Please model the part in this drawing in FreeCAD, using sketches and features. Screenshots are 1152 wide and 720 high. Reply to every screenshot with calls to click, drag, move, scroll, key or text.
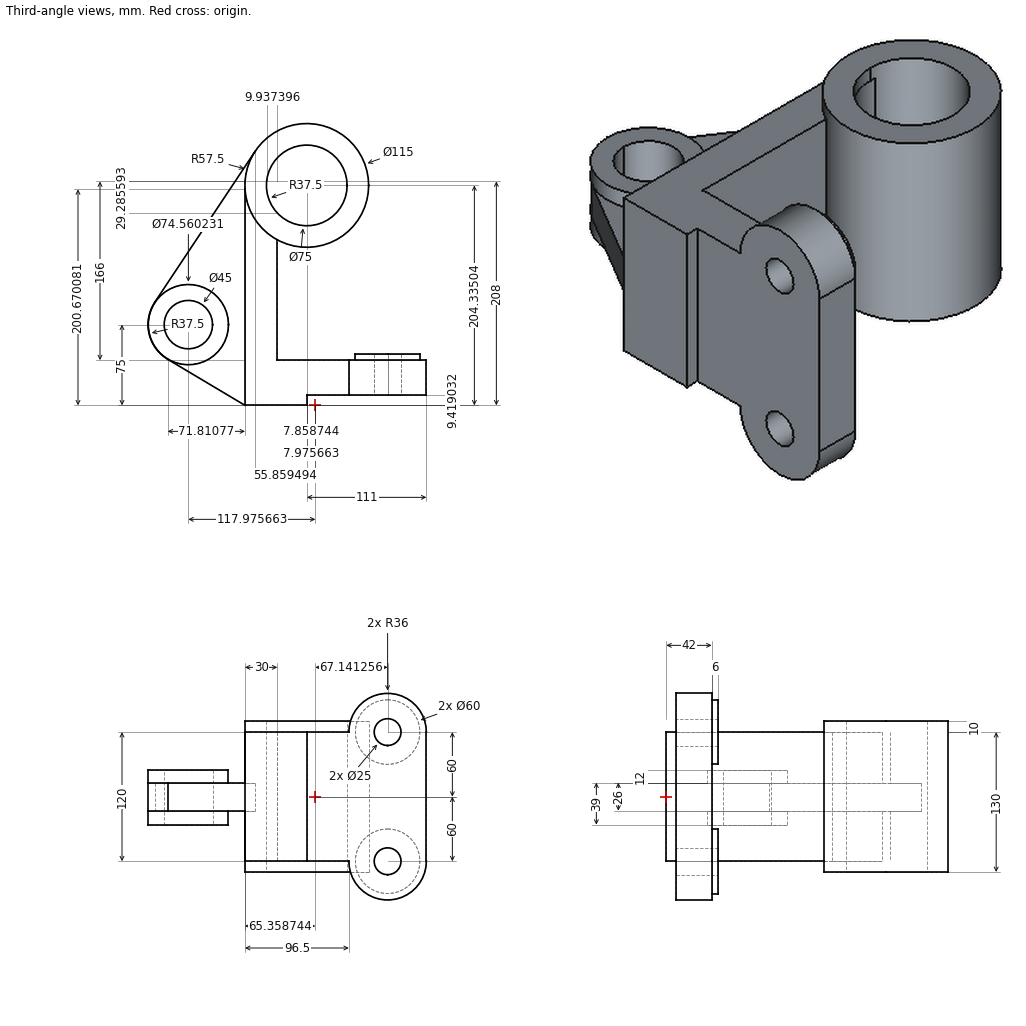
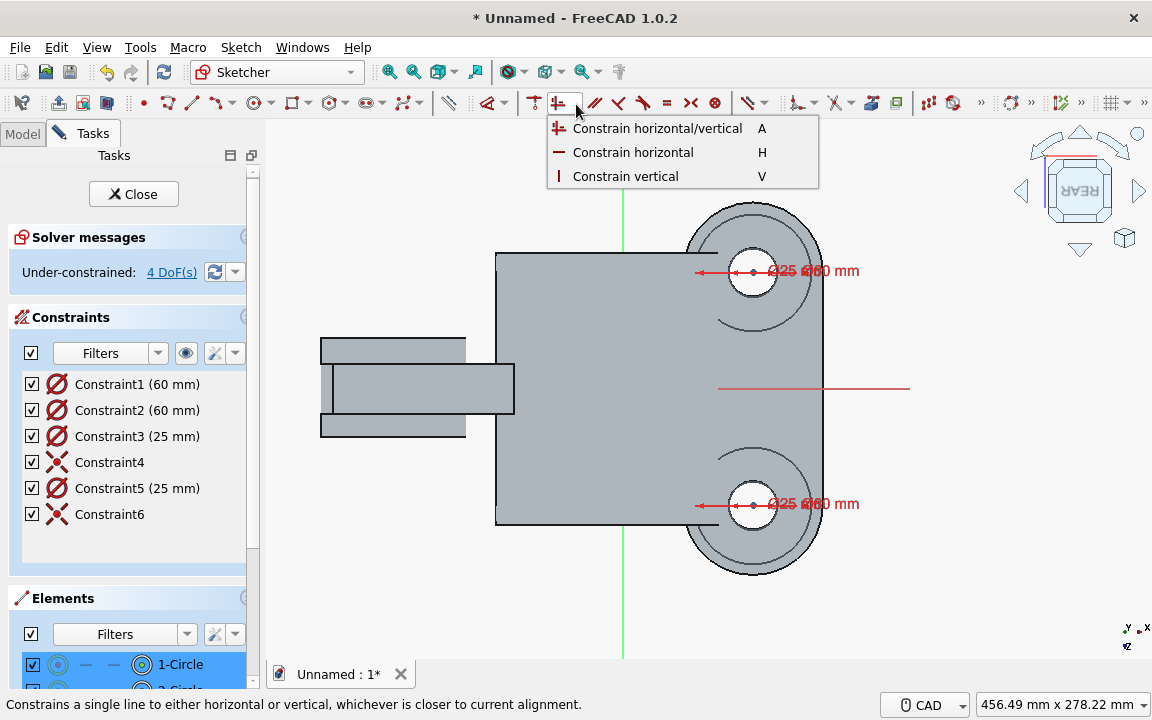
click(683, 176)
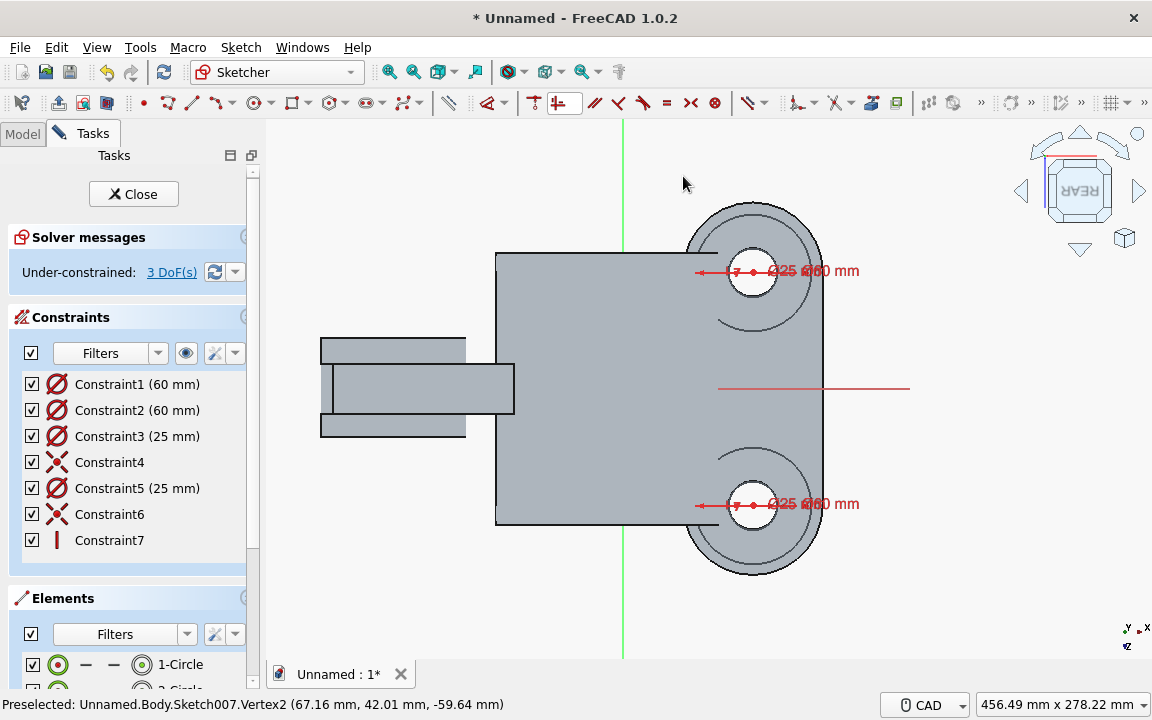
click(488, 104)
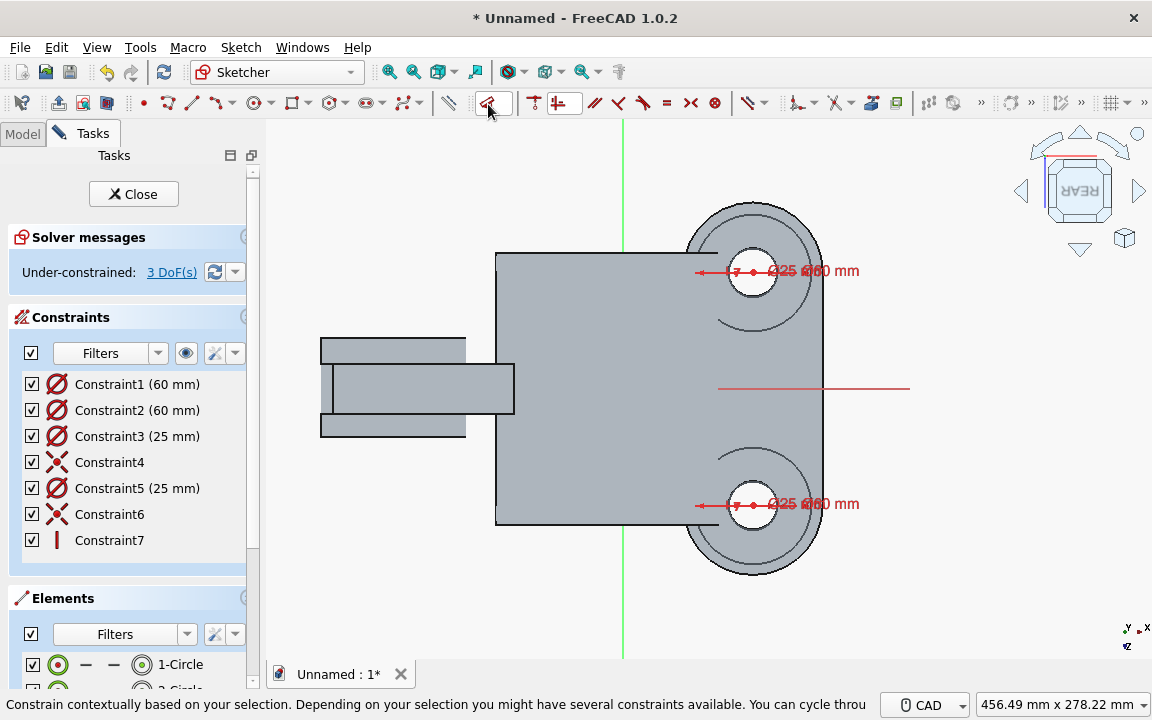
click(753, 506)
click(589, 447)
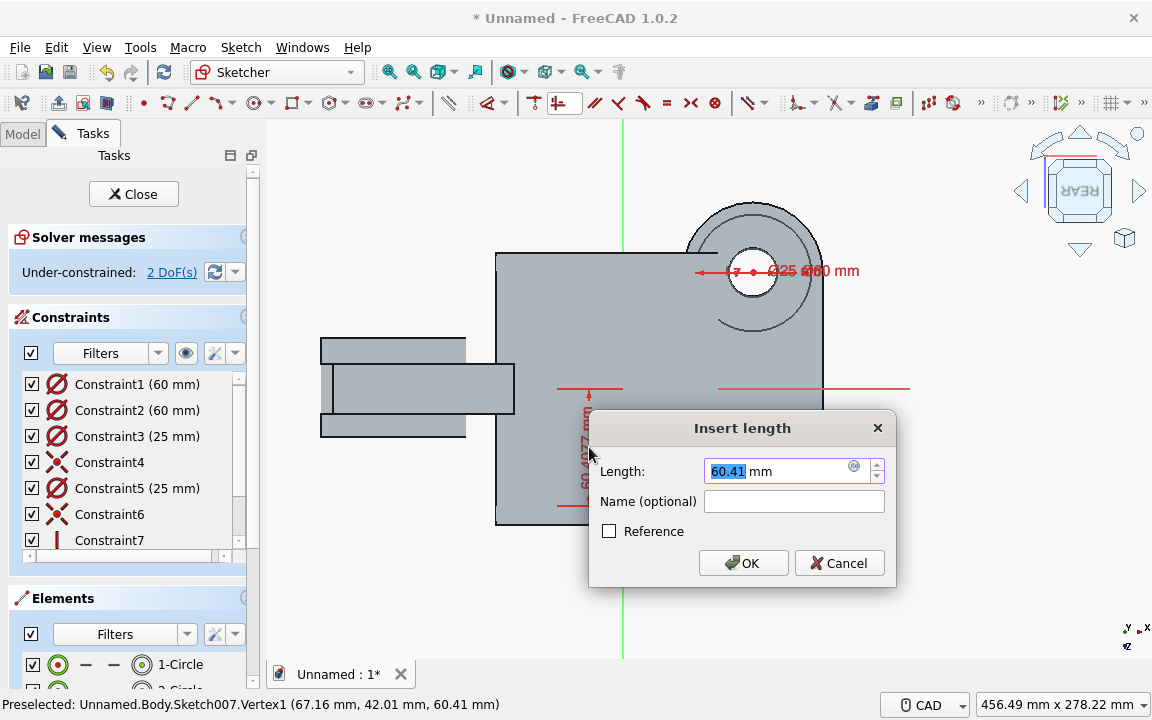
text(60)
key(Return)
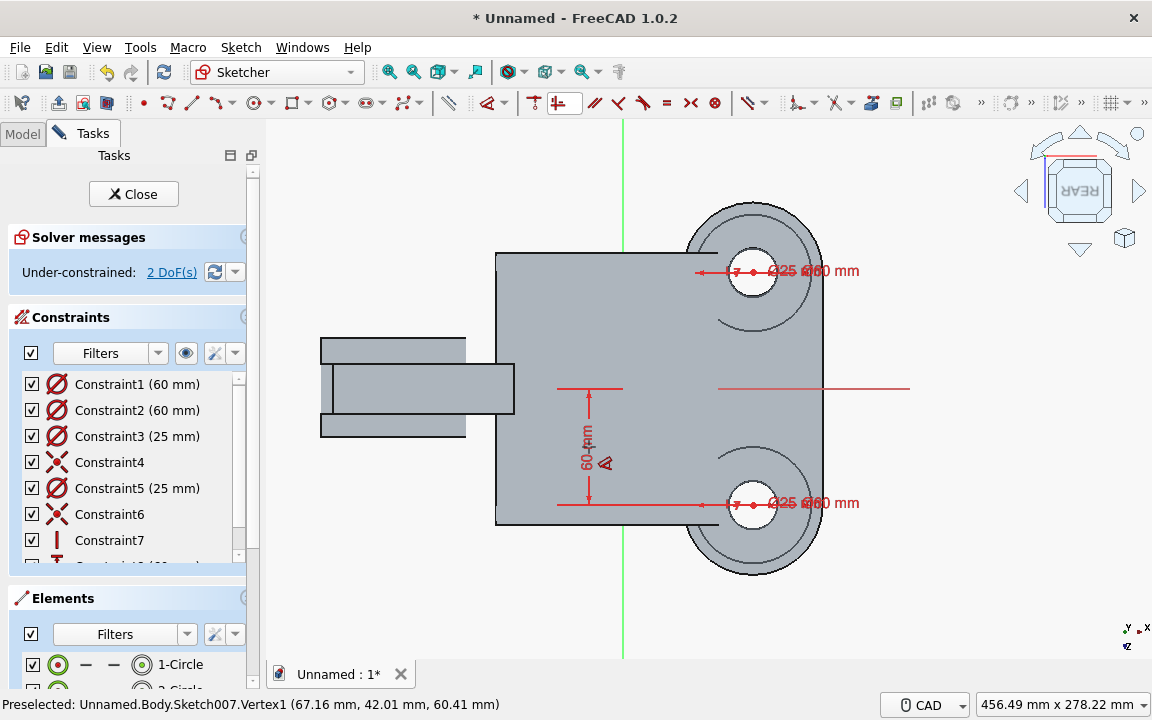
click(753, 273)
click(589, 331)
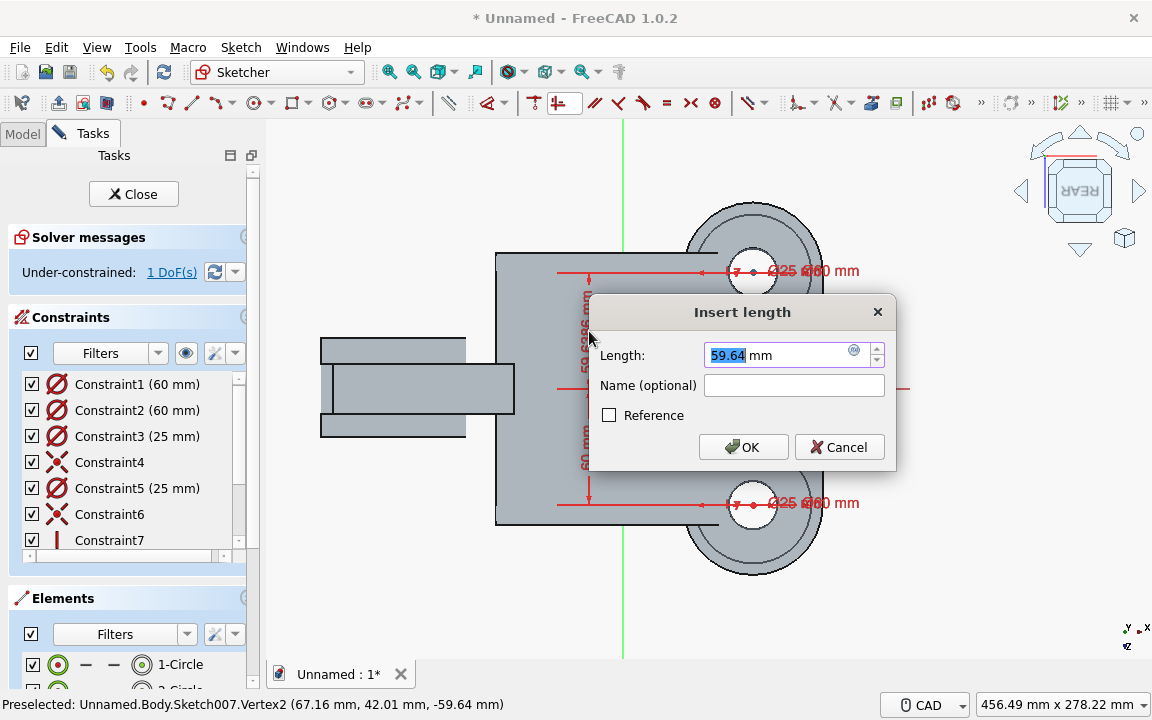
text(60)
key(Return)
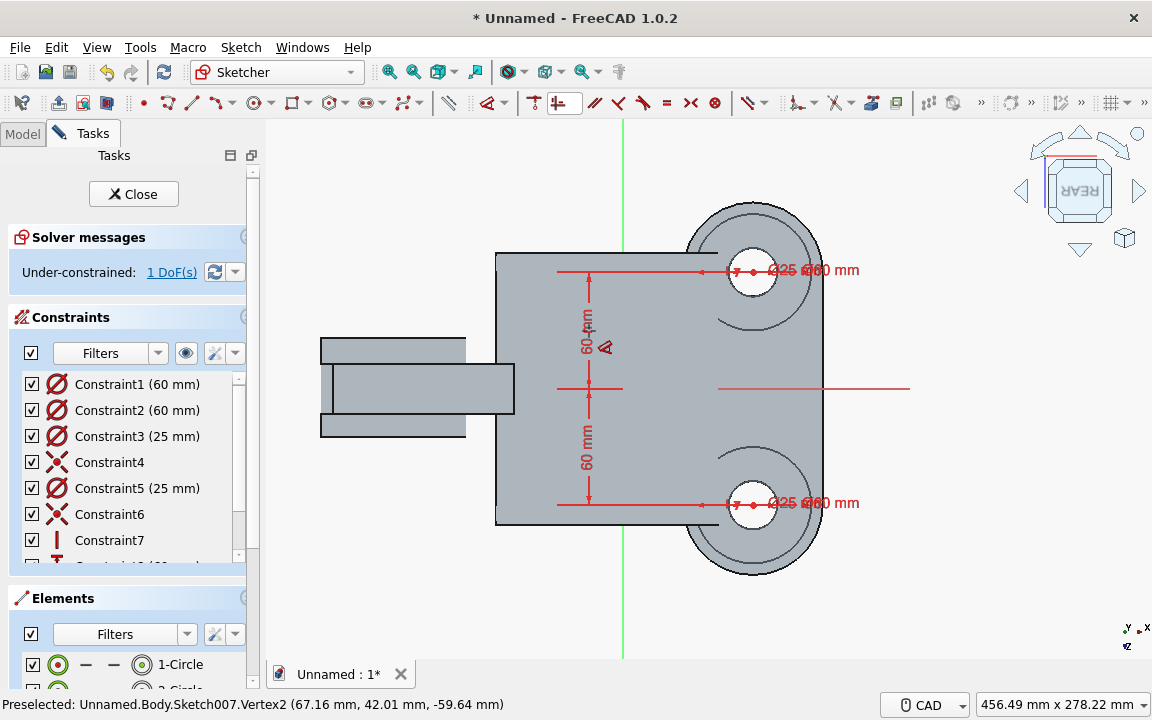
click(753, 505)
click(688, 539)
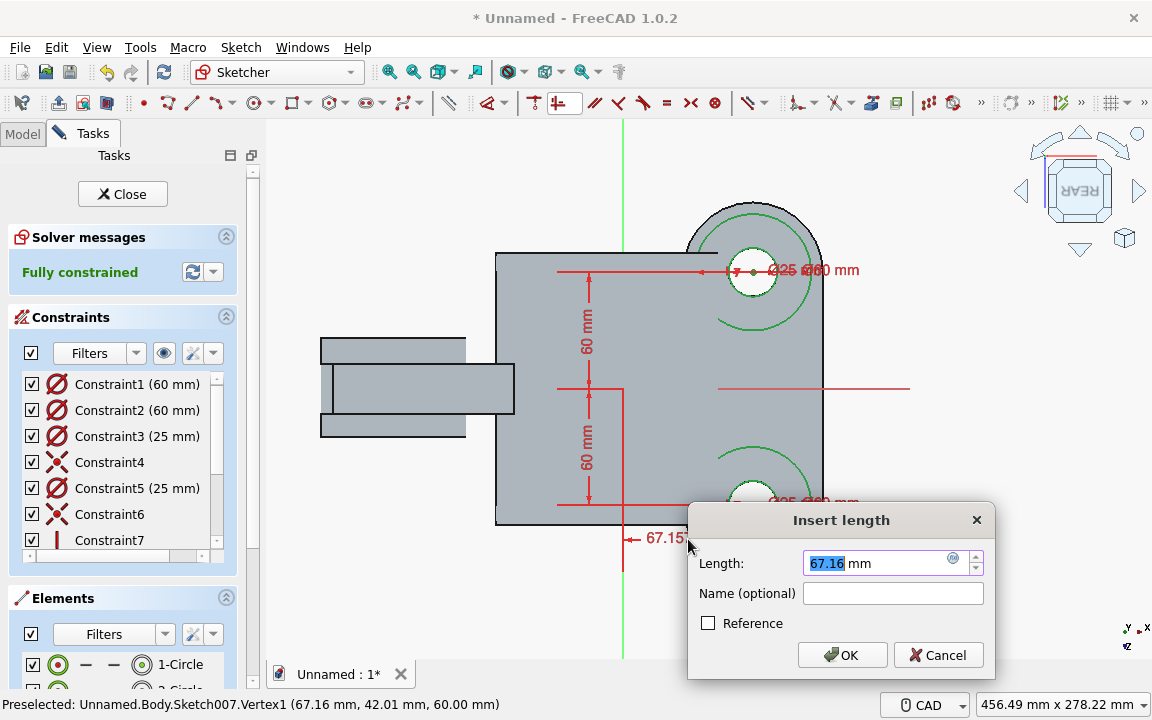
text(67.141256)
key(Return)
key(Escape)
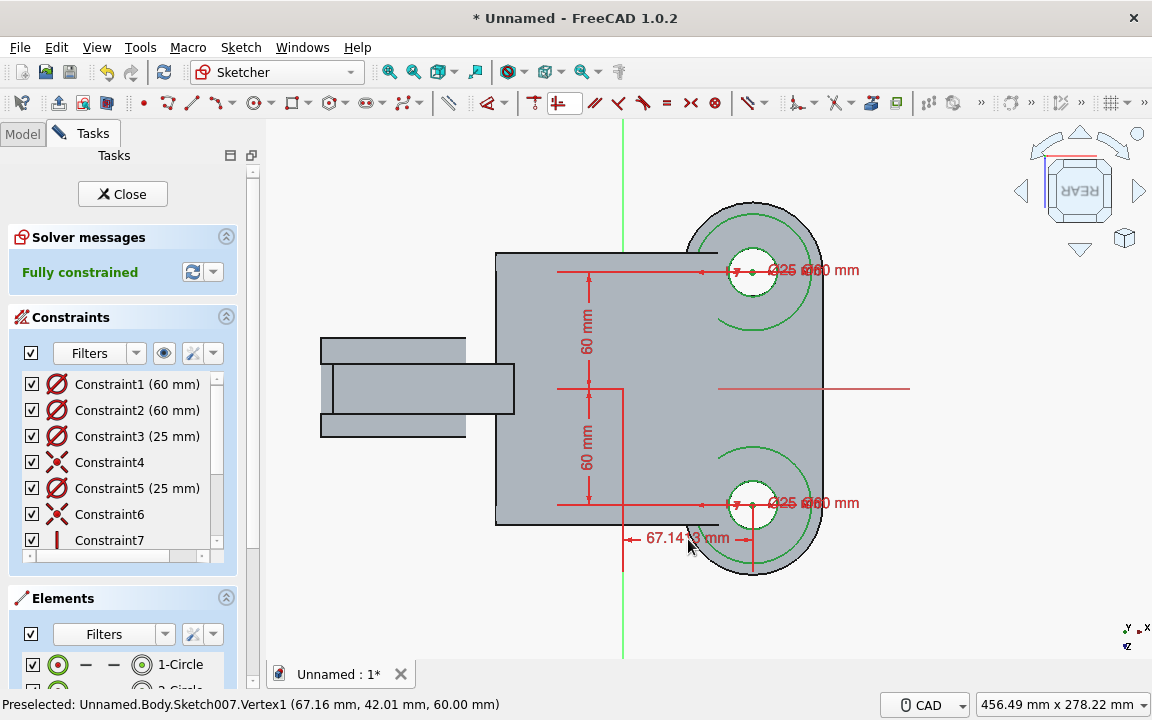
click(123, 194)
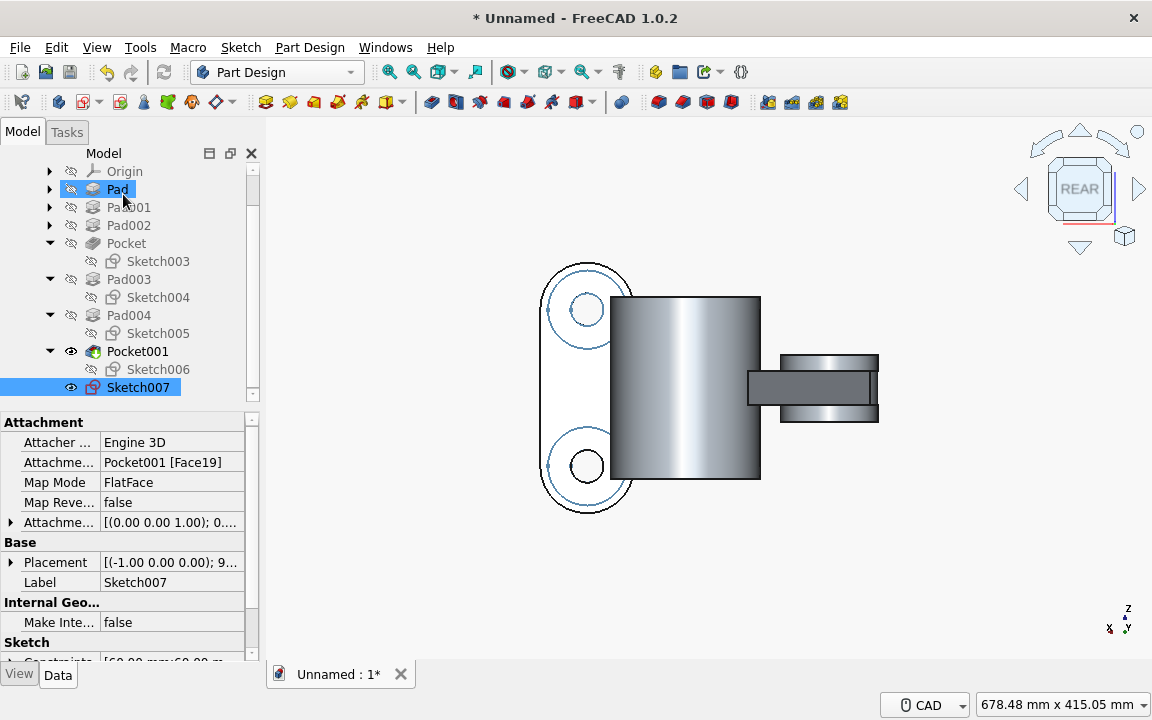
click(266, 102)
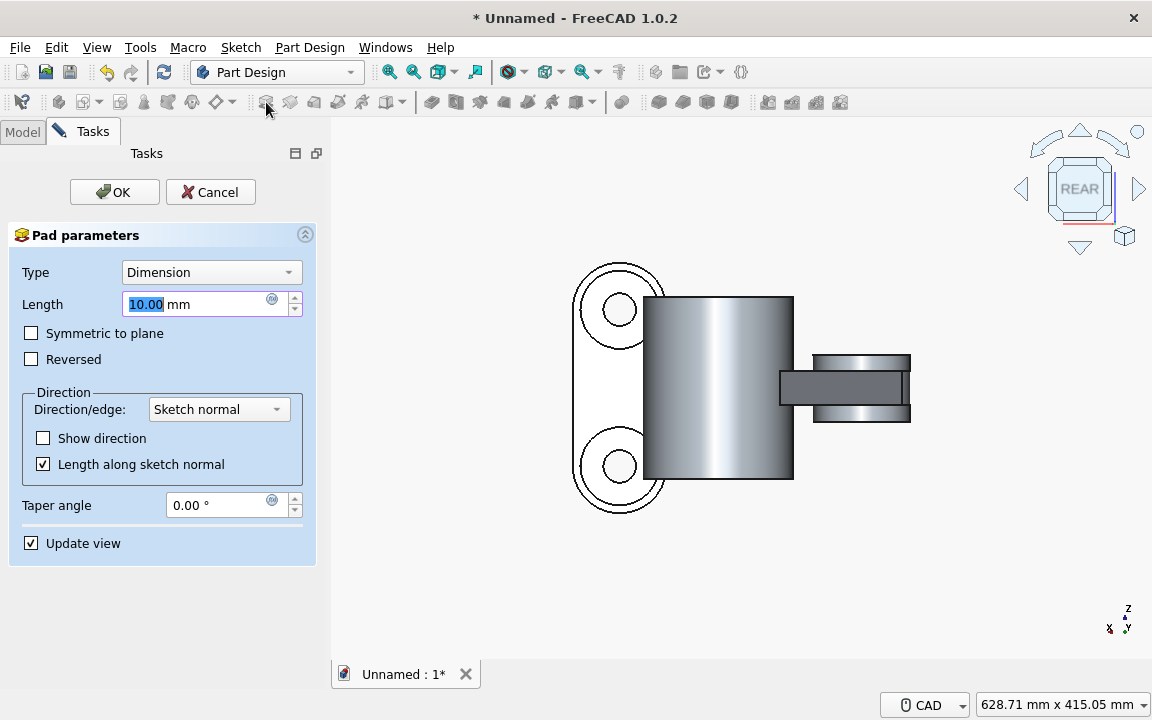
text(6)
key(Tab)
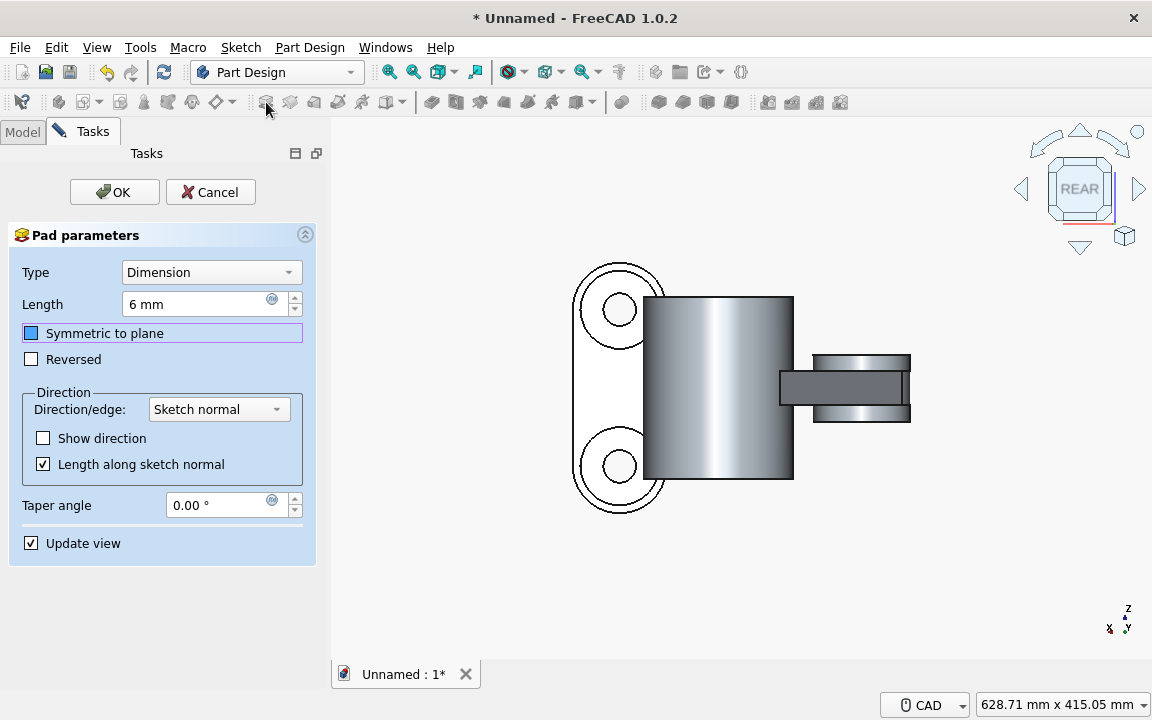
click(115, 192)